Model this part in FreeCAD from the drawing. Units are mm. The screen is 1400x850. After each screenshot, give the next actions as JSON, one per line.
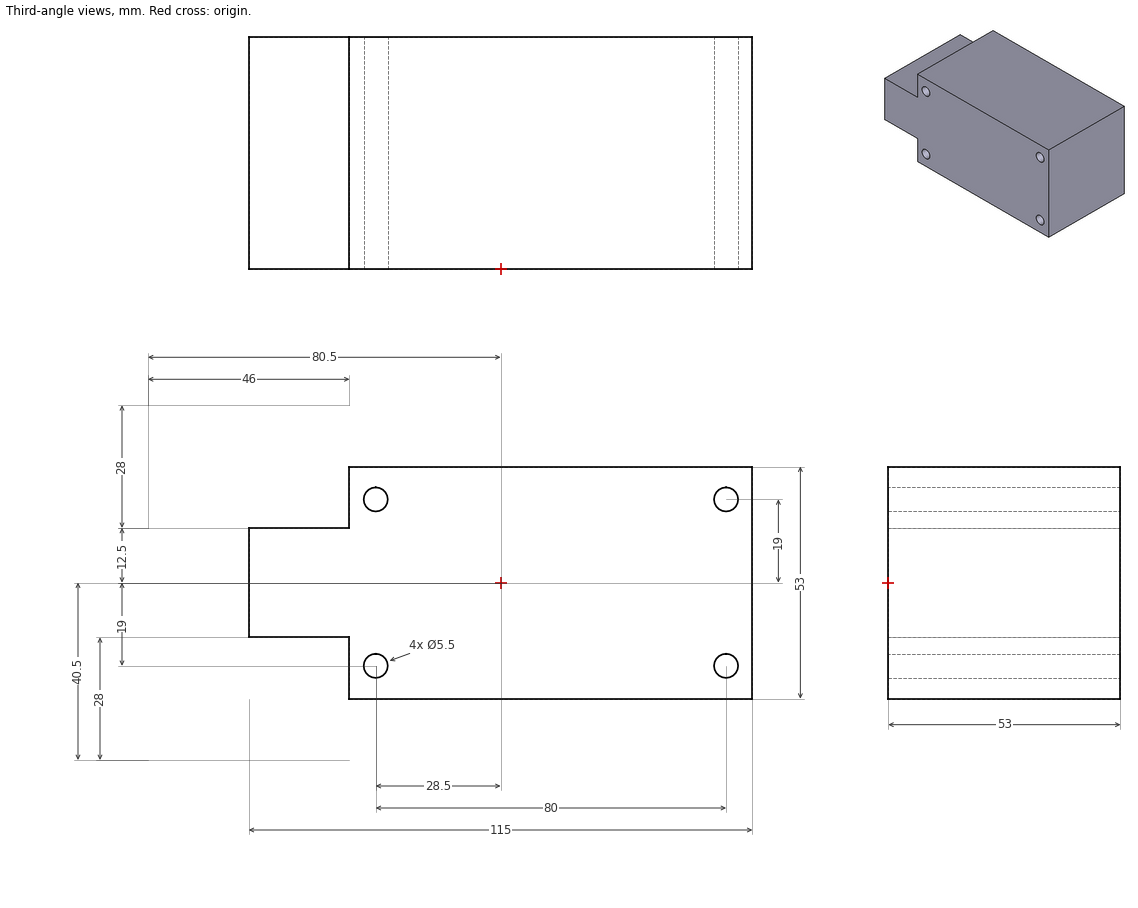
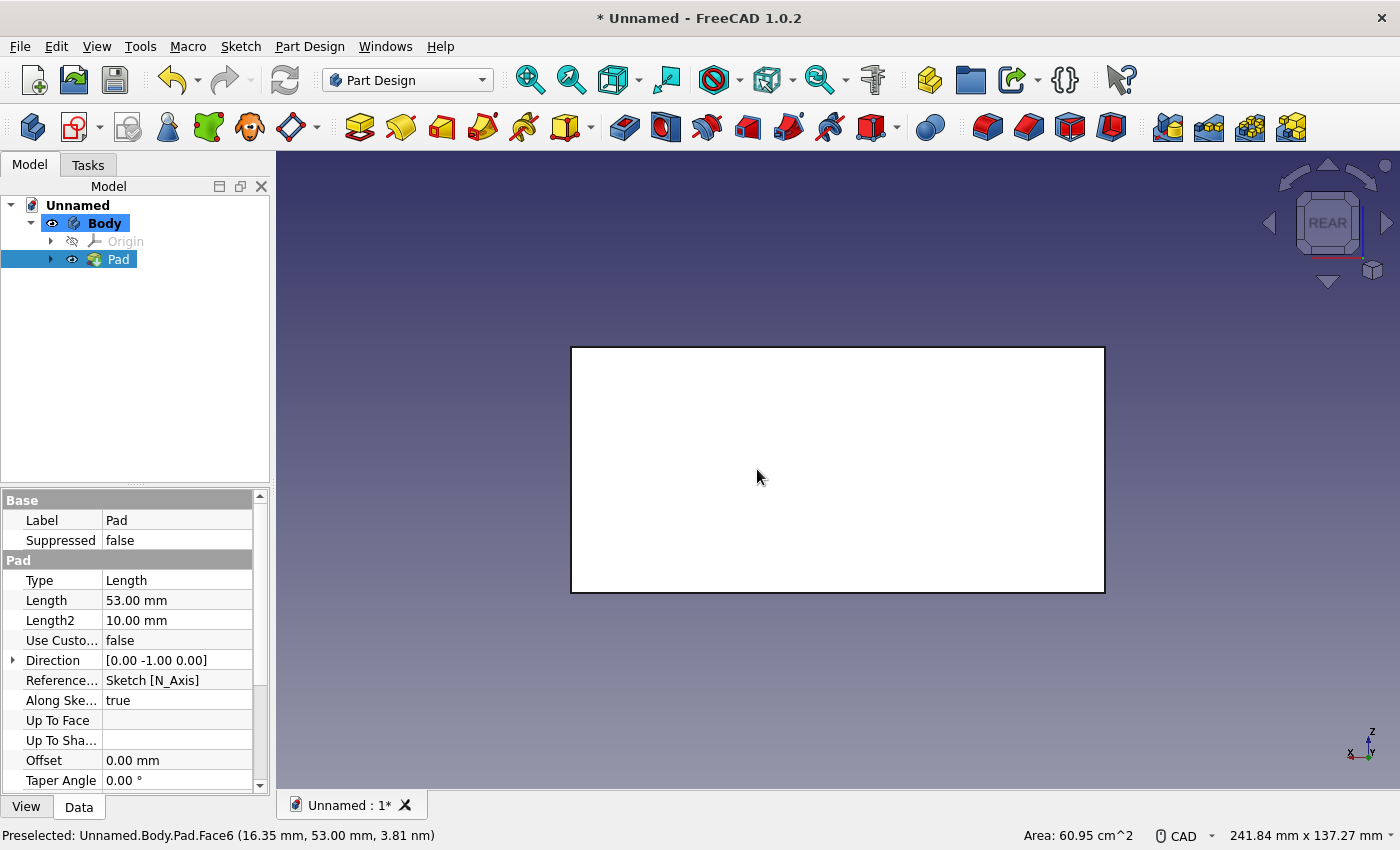
{"action": "left_click", "coordinate": [74, 128]}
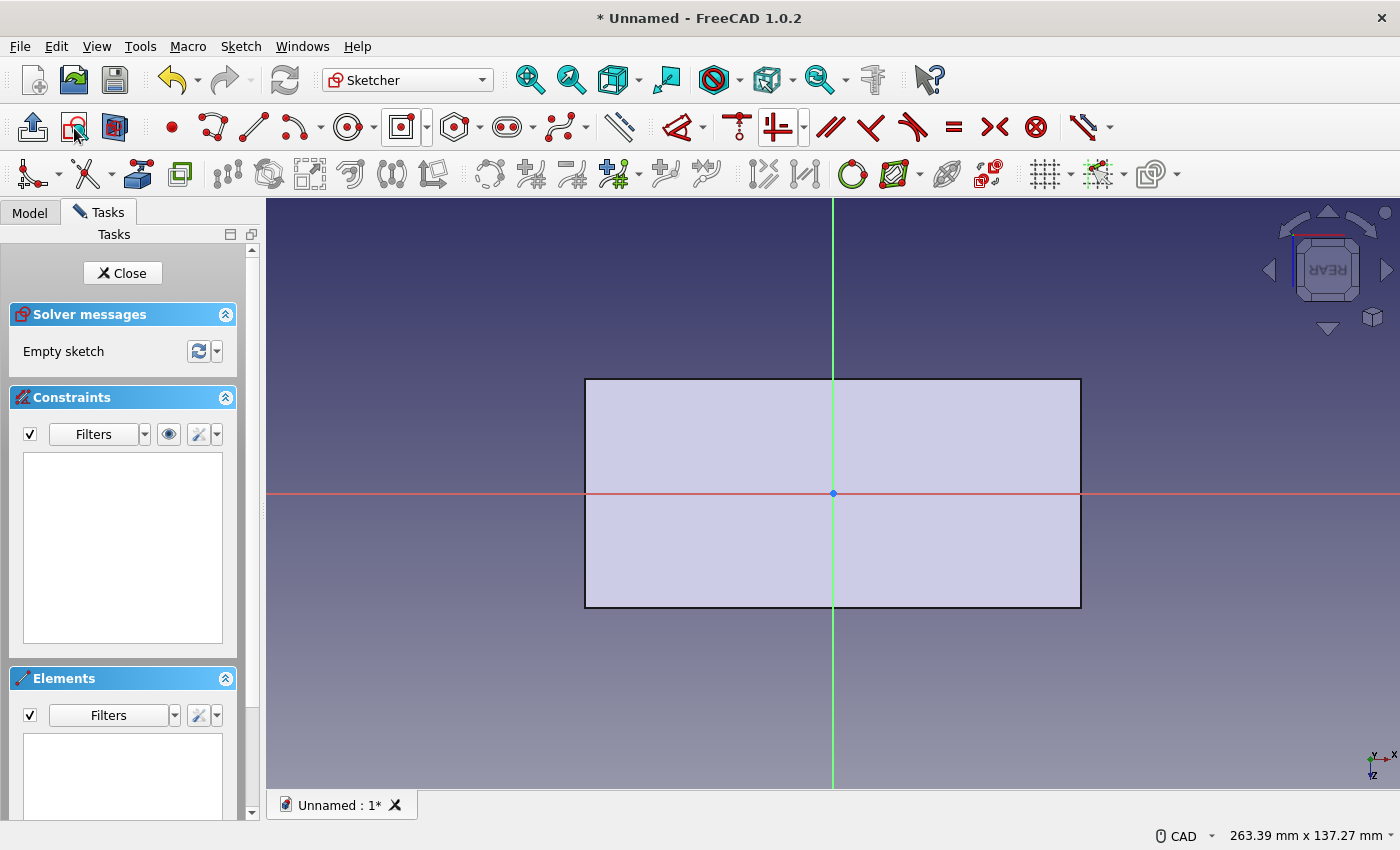
{"action": "key", "text": "g r"}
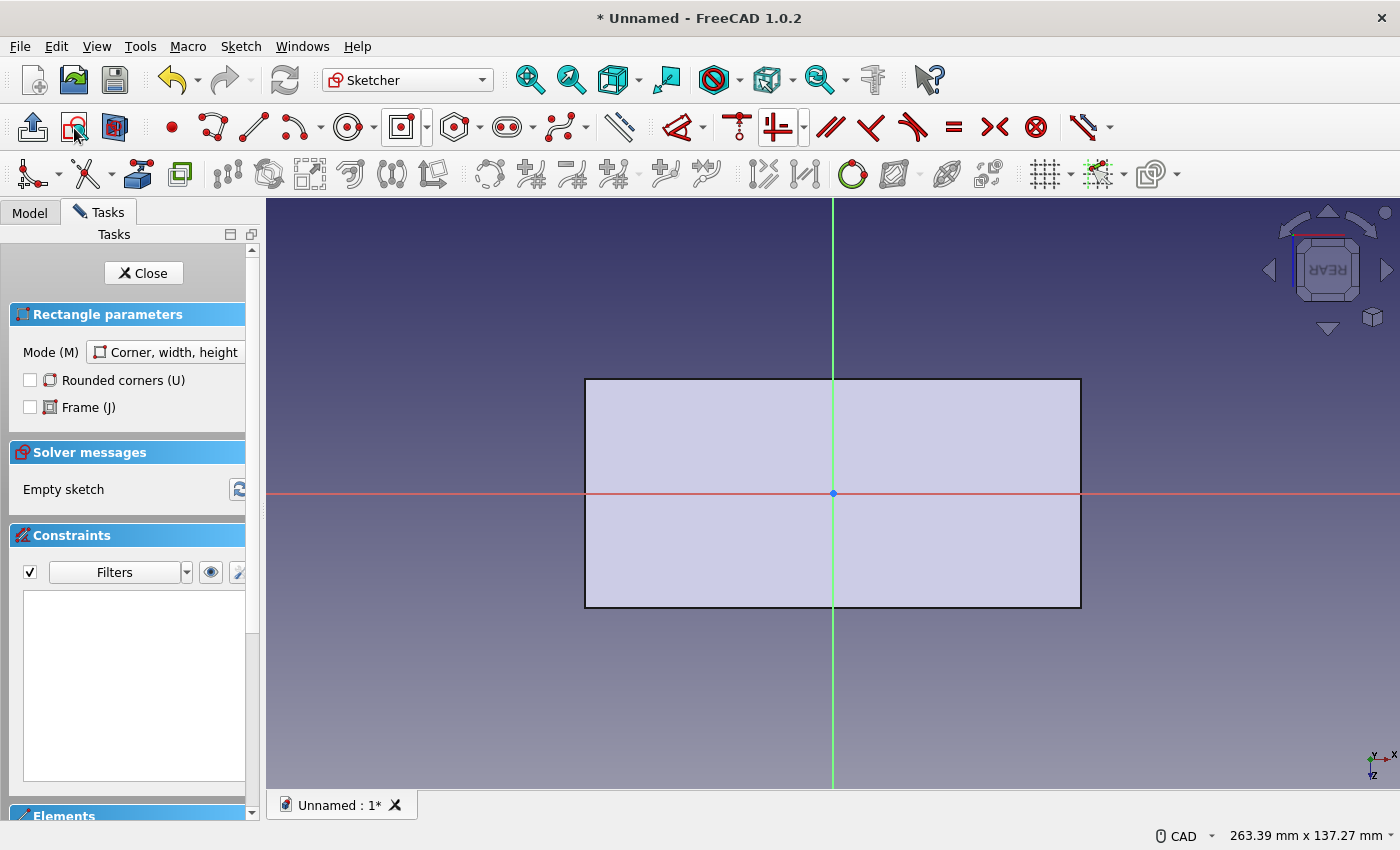
{"action": "left_click", "coordinate": [486, 547]}
{"action": "mouse_move", "coordinate": [684, 668]}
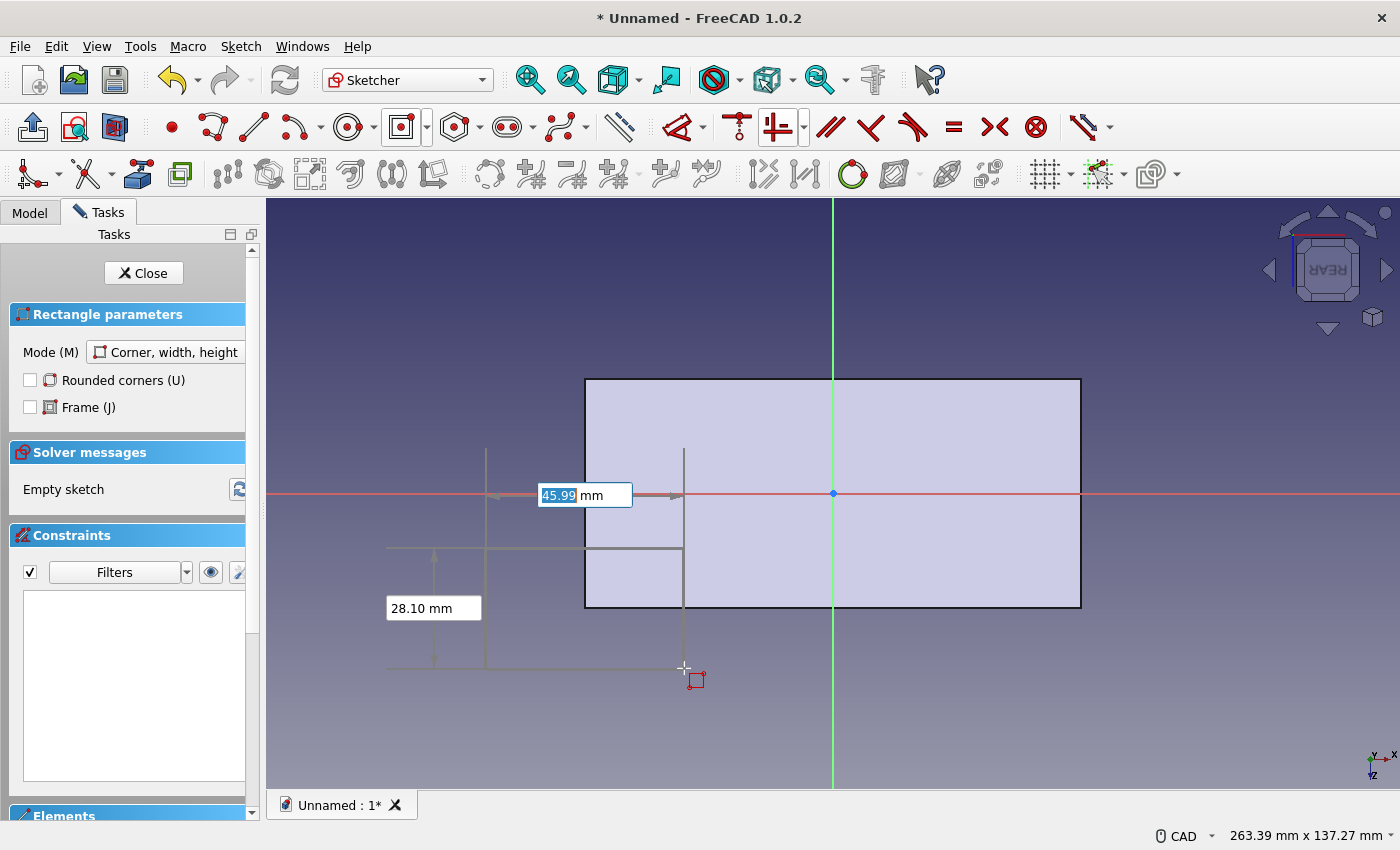
{"action": "type", "text": "46"}
{"action": "key", "text": "Tab"}
{"action": "type", "text": "28"}
{"action": "key", "text": "Return"}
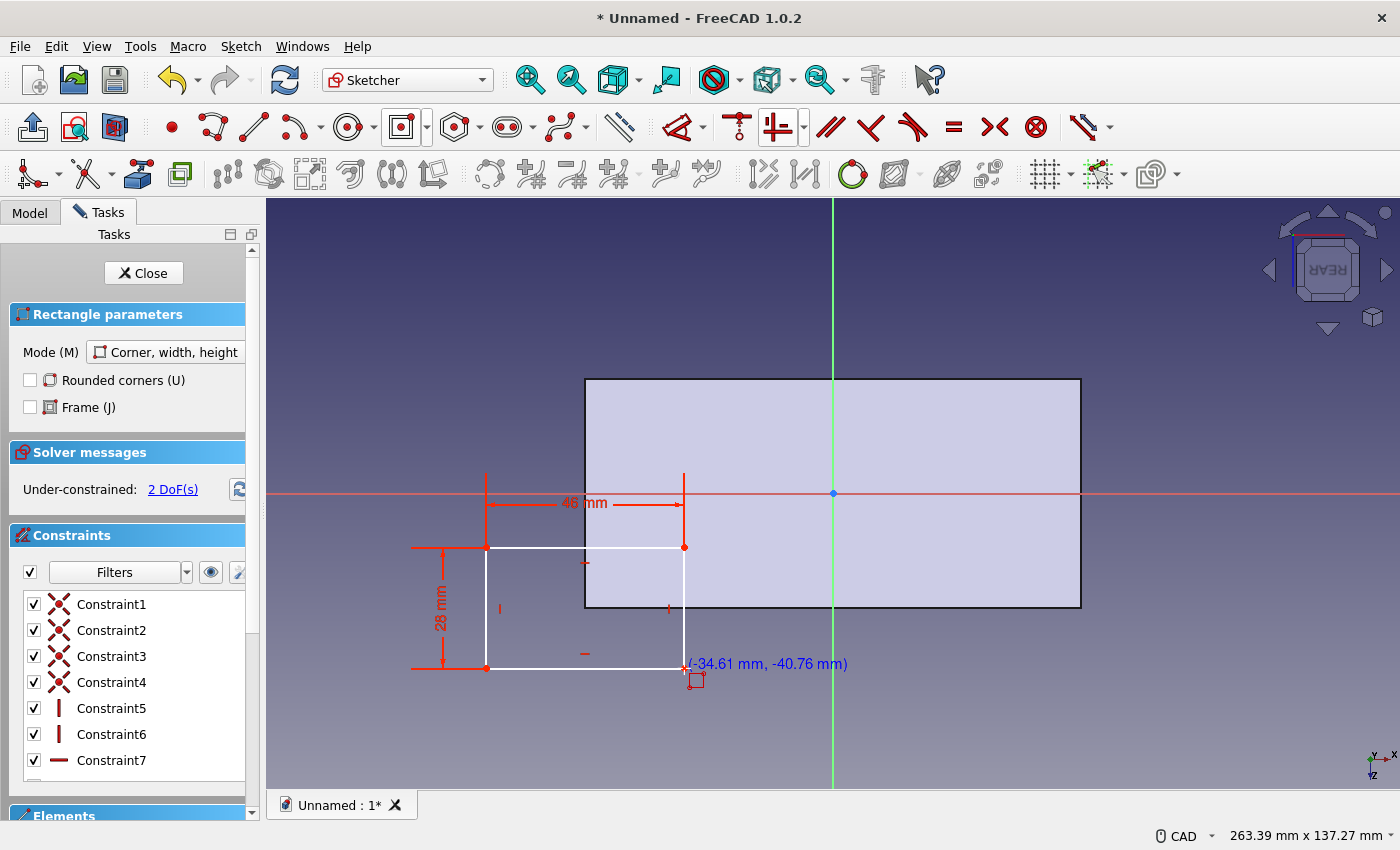
{"action": "left_click", "coordinate": [486, 319]}
{"action": "mouse_move", "coordinate": [684, 440]}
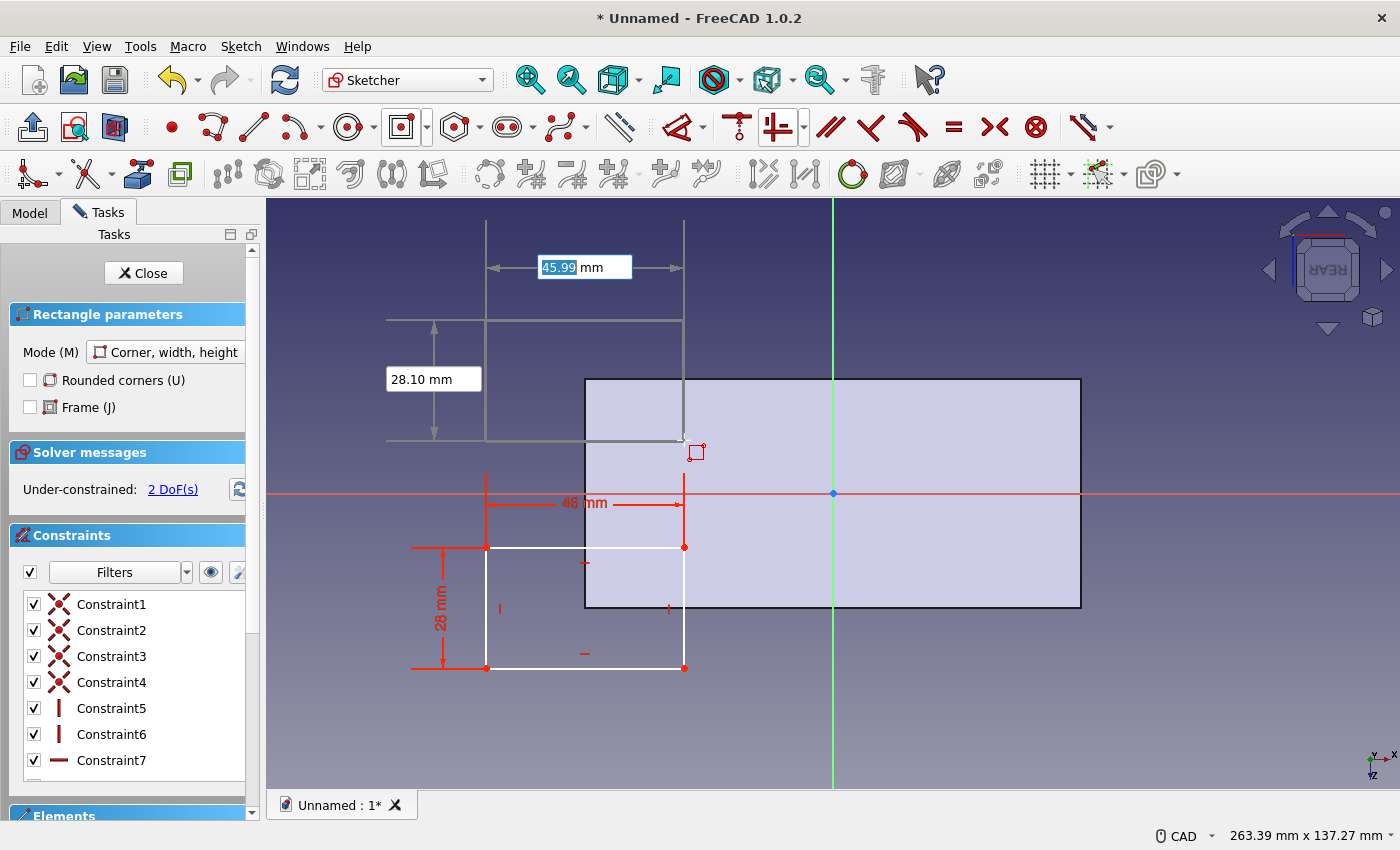
{"action": "type", "text": "46"}
{"action": "key", "text": "Tab"}
{"action": "type", "text": "28"}
{"action": "key", "text": "Return"}
{"action": "key", "text": "Escape"}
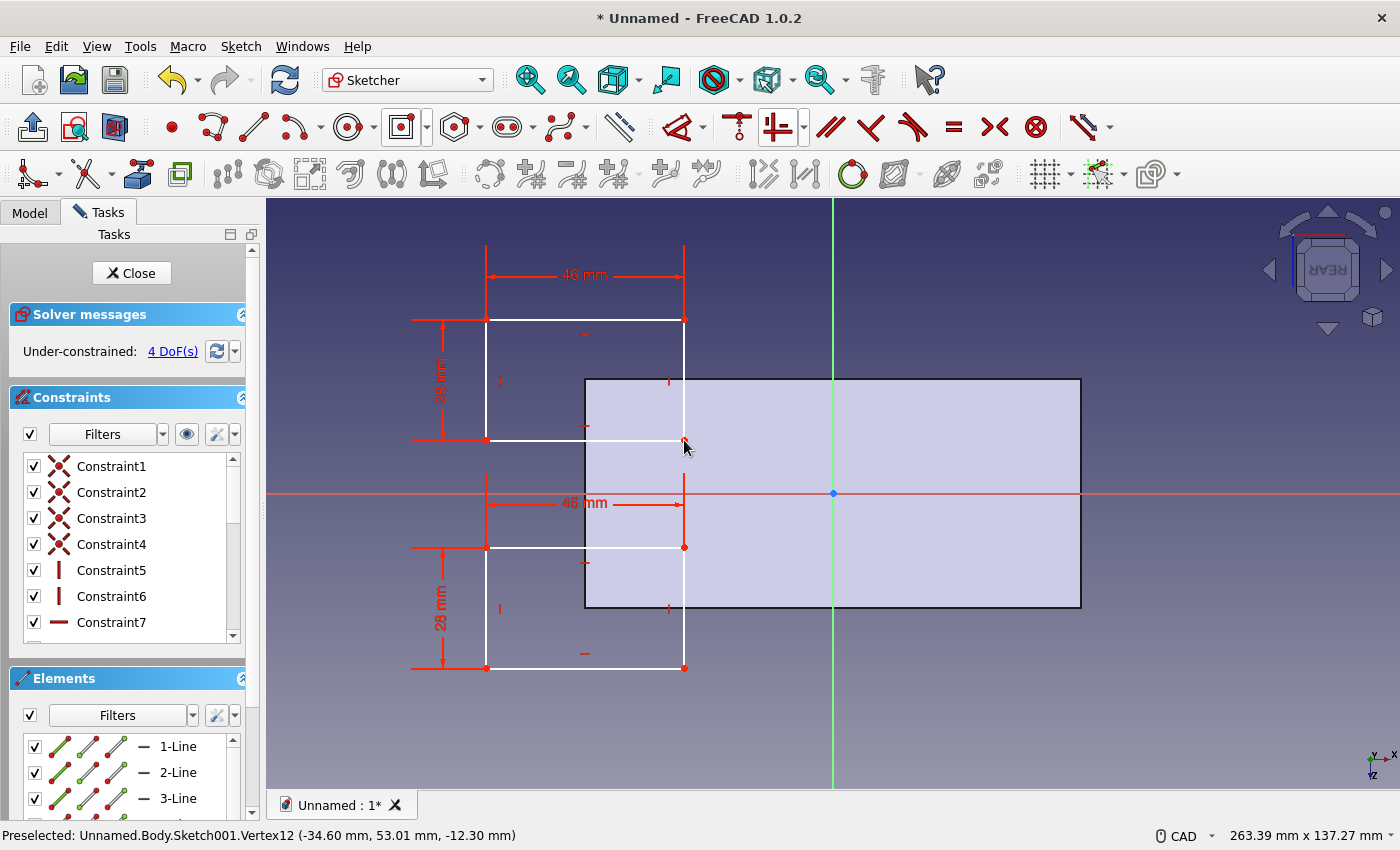
{"action": "left_click", "coordinate": [676, 128]}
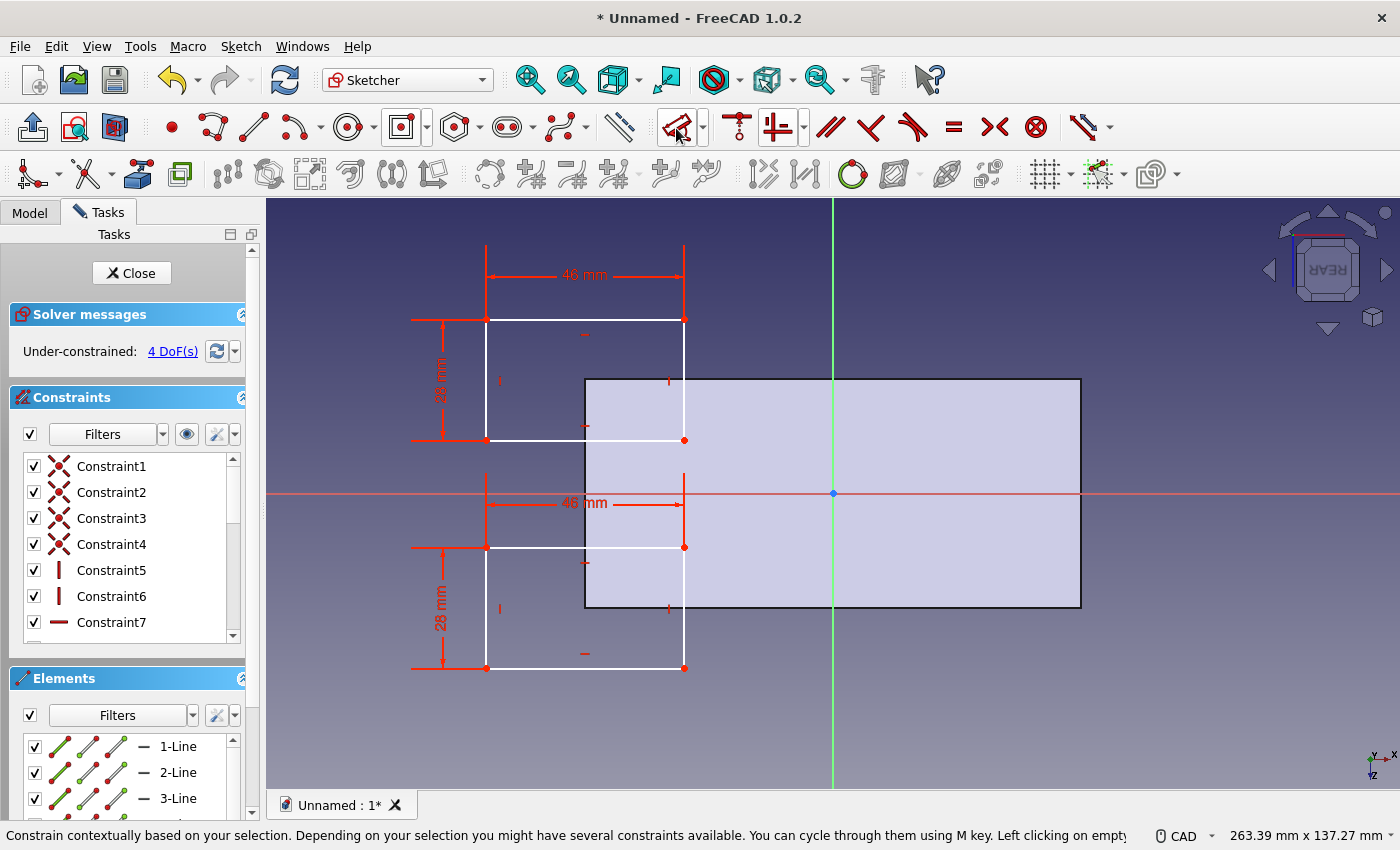
{"action": "left_click", "coordinate": [486, 548]}
{"action": "left_click", "coordinate": [659, 582]}